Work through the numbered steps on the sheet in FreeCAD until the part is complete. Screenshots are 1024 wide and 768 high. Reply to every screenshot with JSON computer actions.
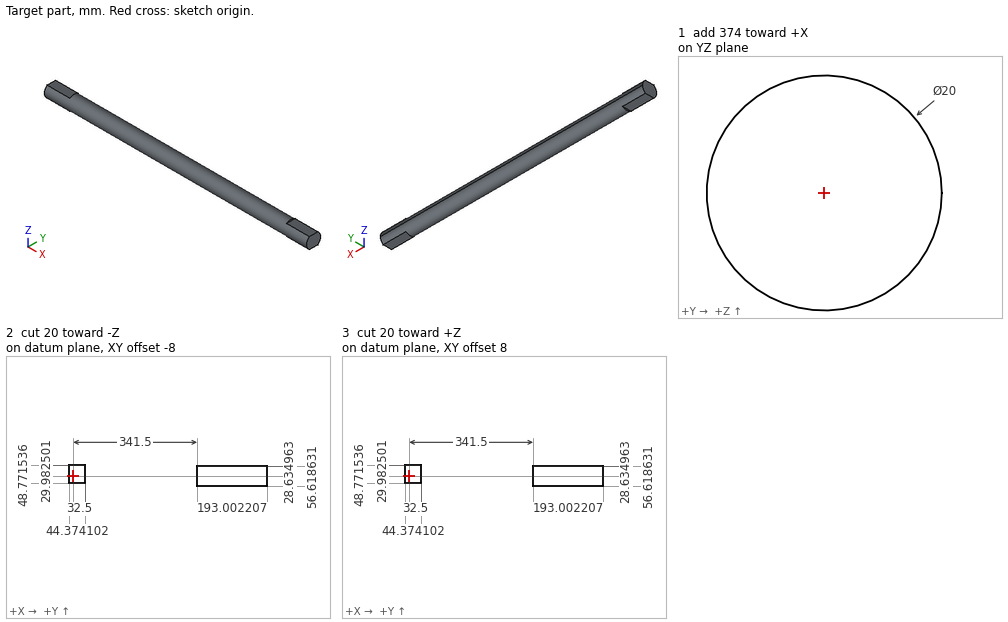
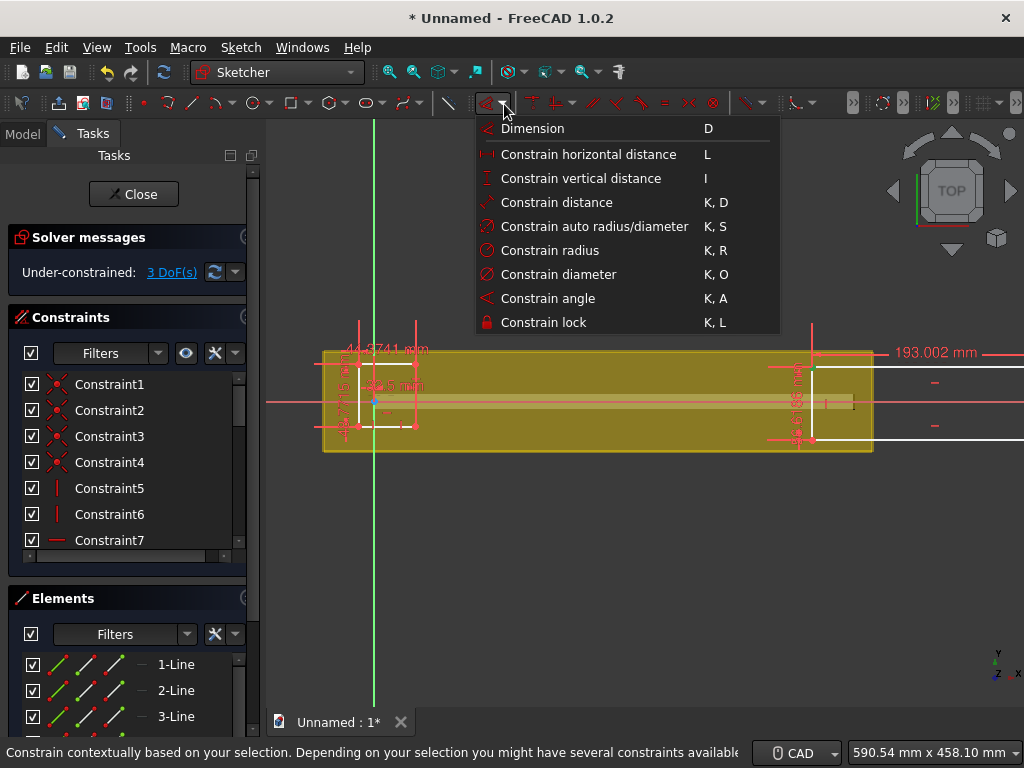
{"action": "left_click", "coordinate": [628, 154]}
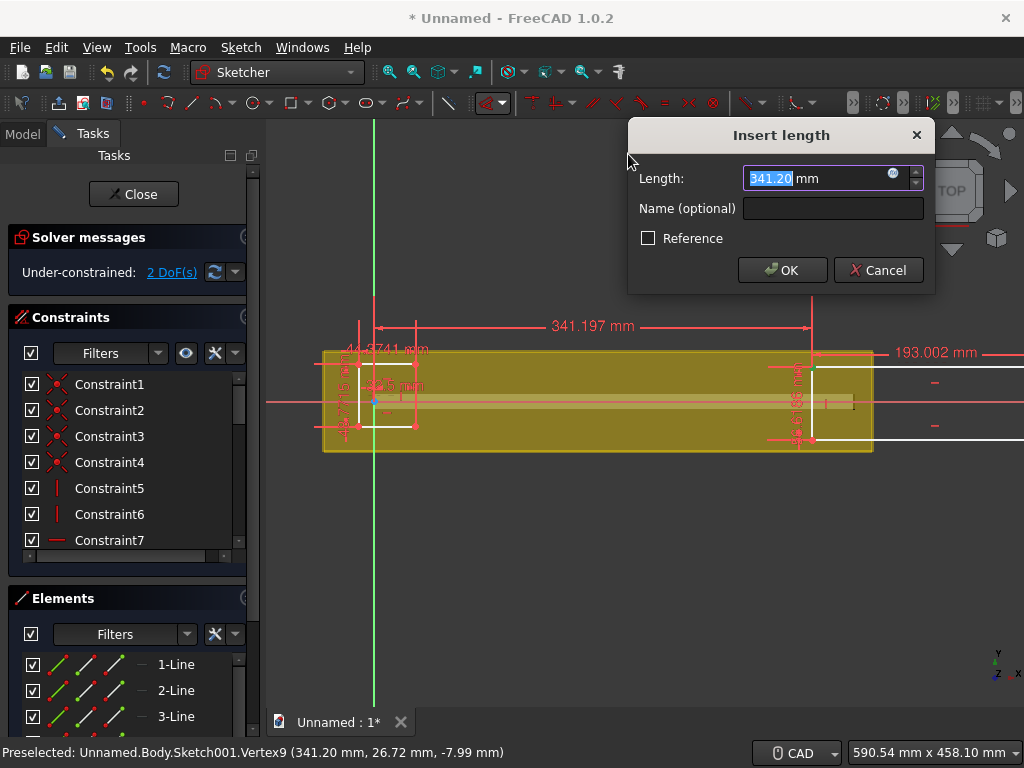
{"action": "type", "text": "341.5"}
{"action": "key", "text": "Return"}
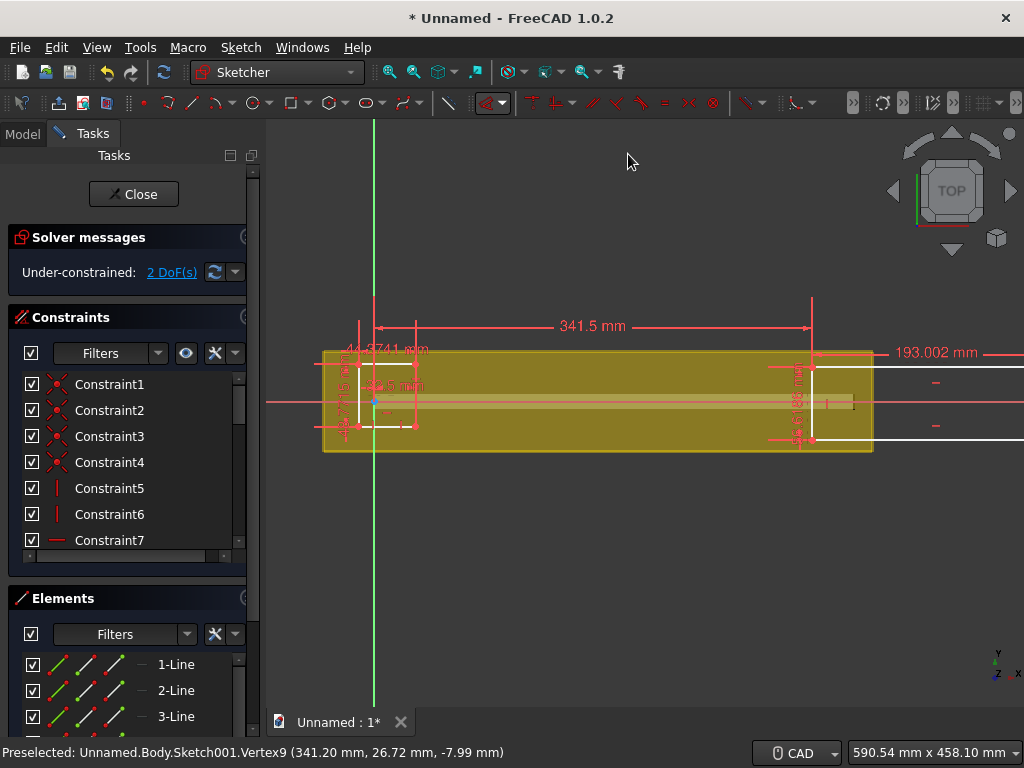
{"action": "left_click", "coordinate": [359, 364]}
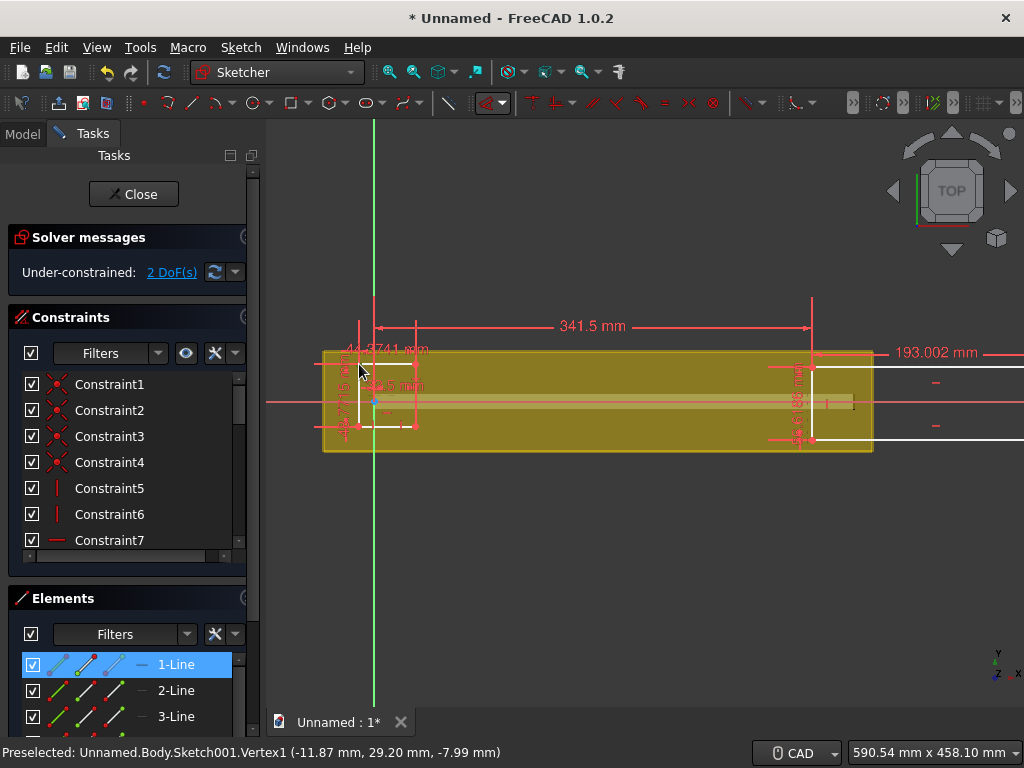
{"action": "left_click", "coordinate": [504, 104]}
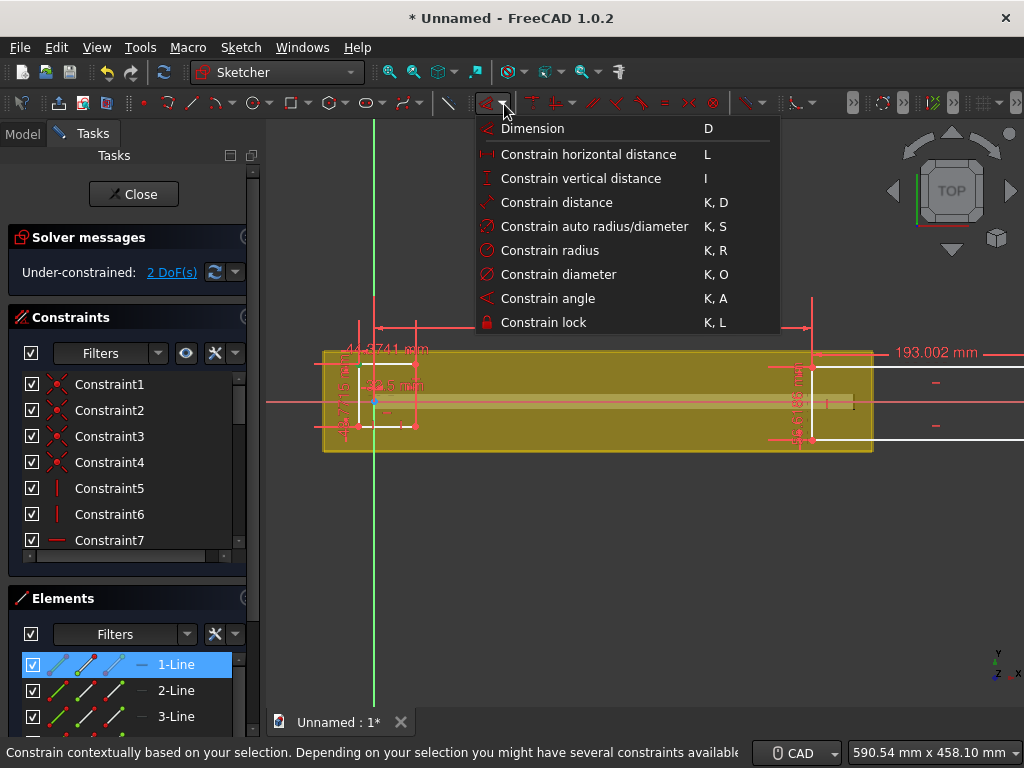
{"action": "left_click", "coordinate": [628, 178]}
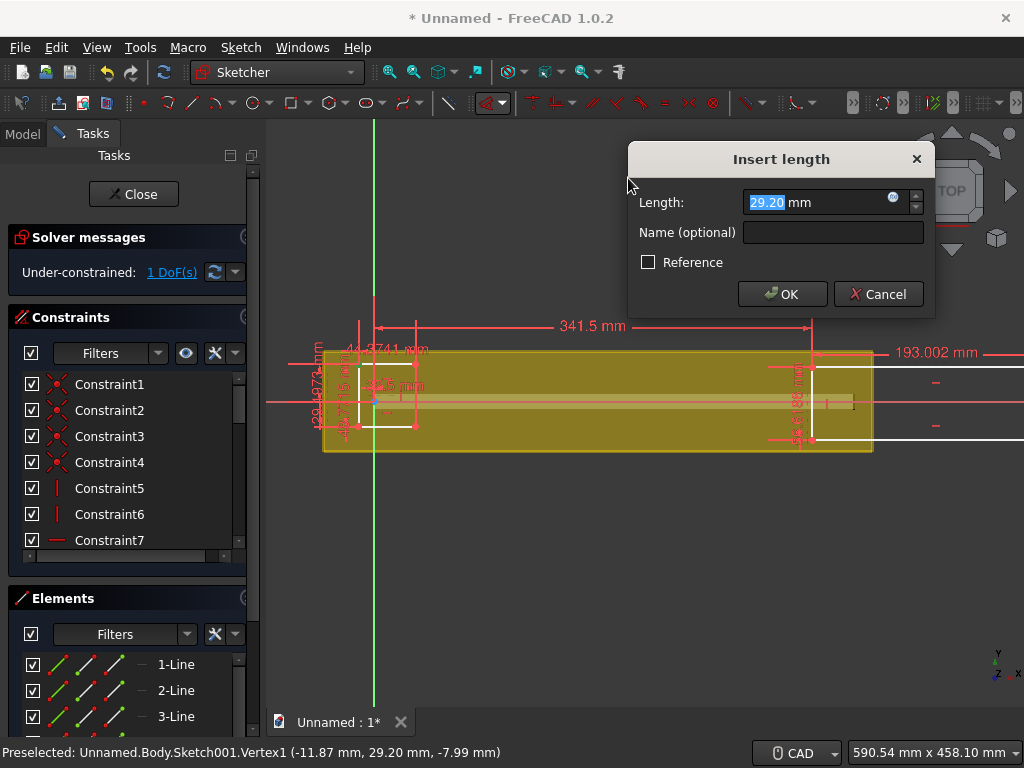
{"action": "type", "text": "29.982501"}
{"action": "key", "text": "Return"}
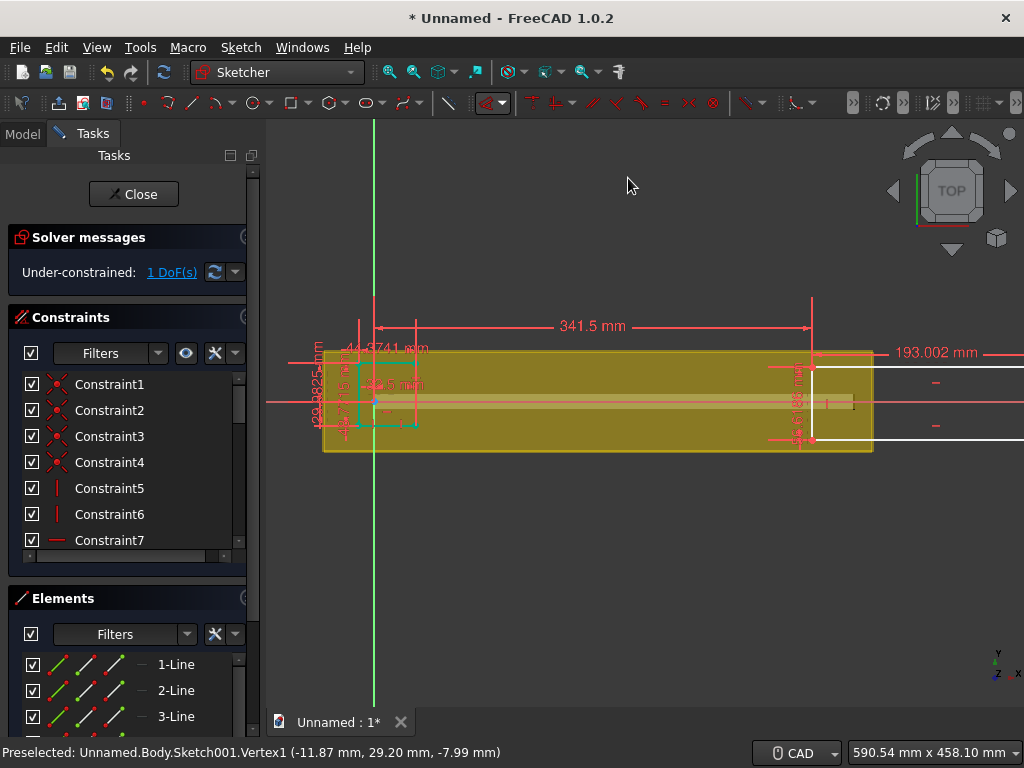
{"action": "left_click", "coordinate": [812, 367]}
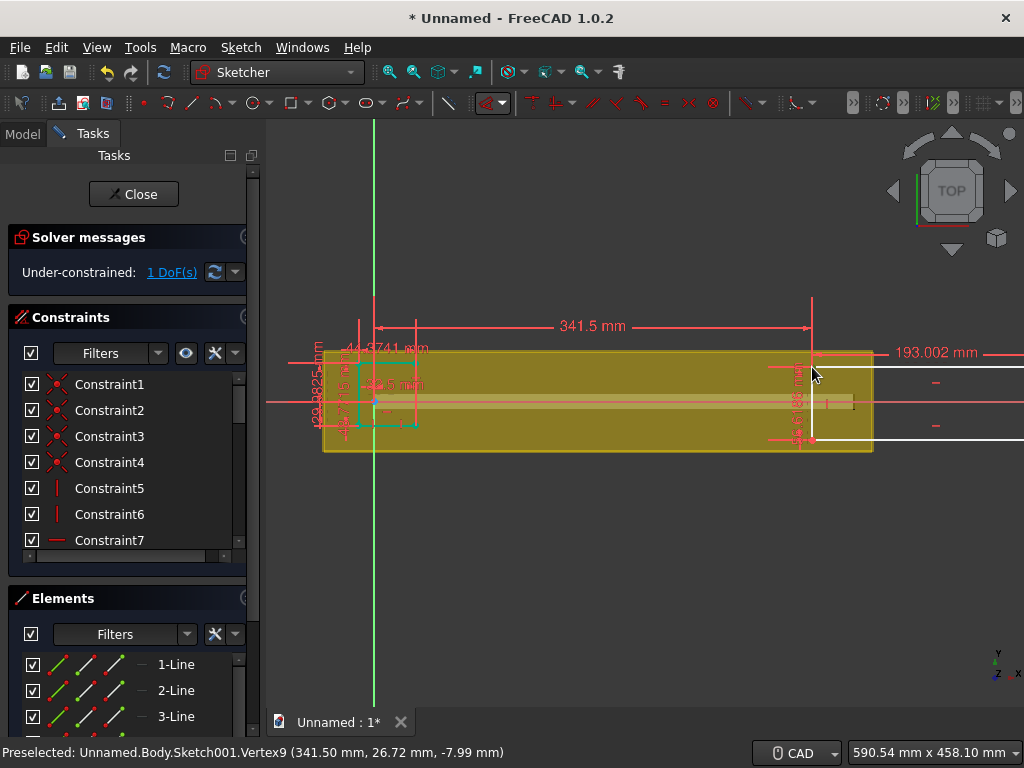
{"action": "key", "text": "i"}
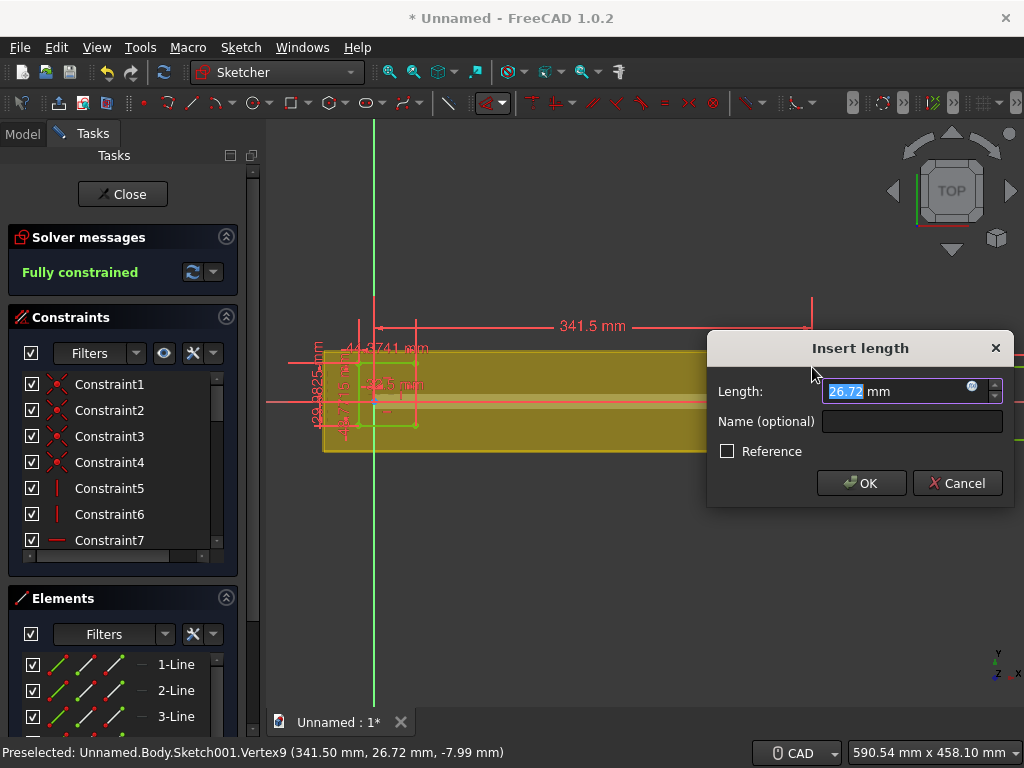
{"action": "type", "text": "28.634963"}
{"action": "key", "text": "Return"}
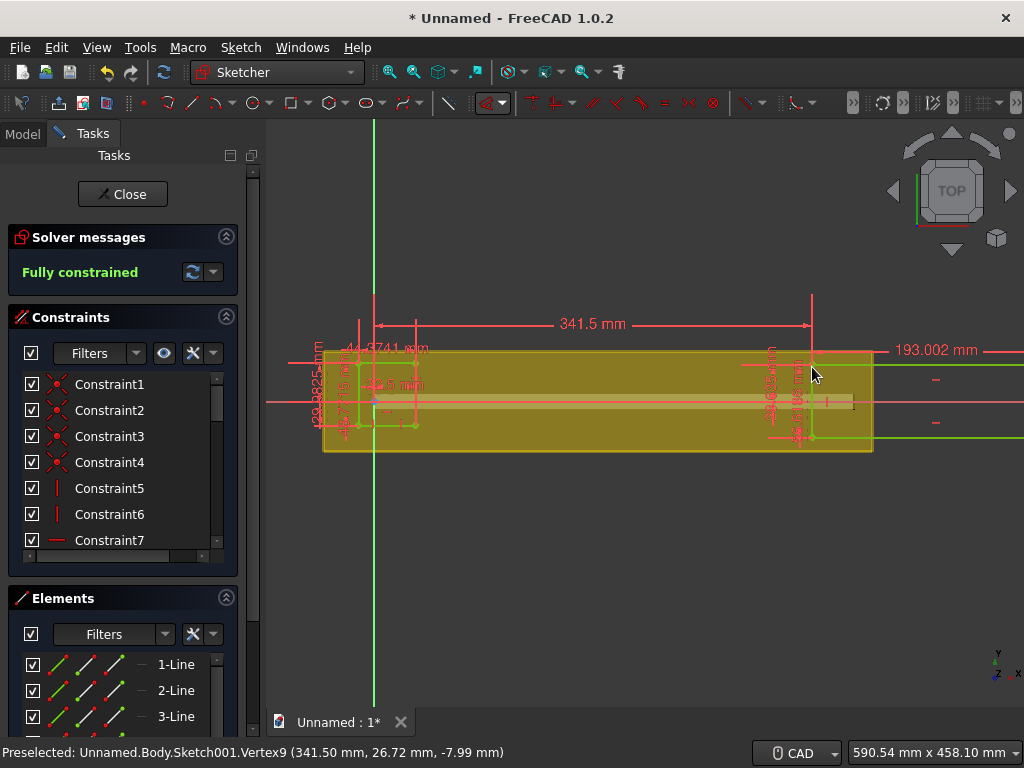
{"action": "left_click", "coordinate": [123, 194]}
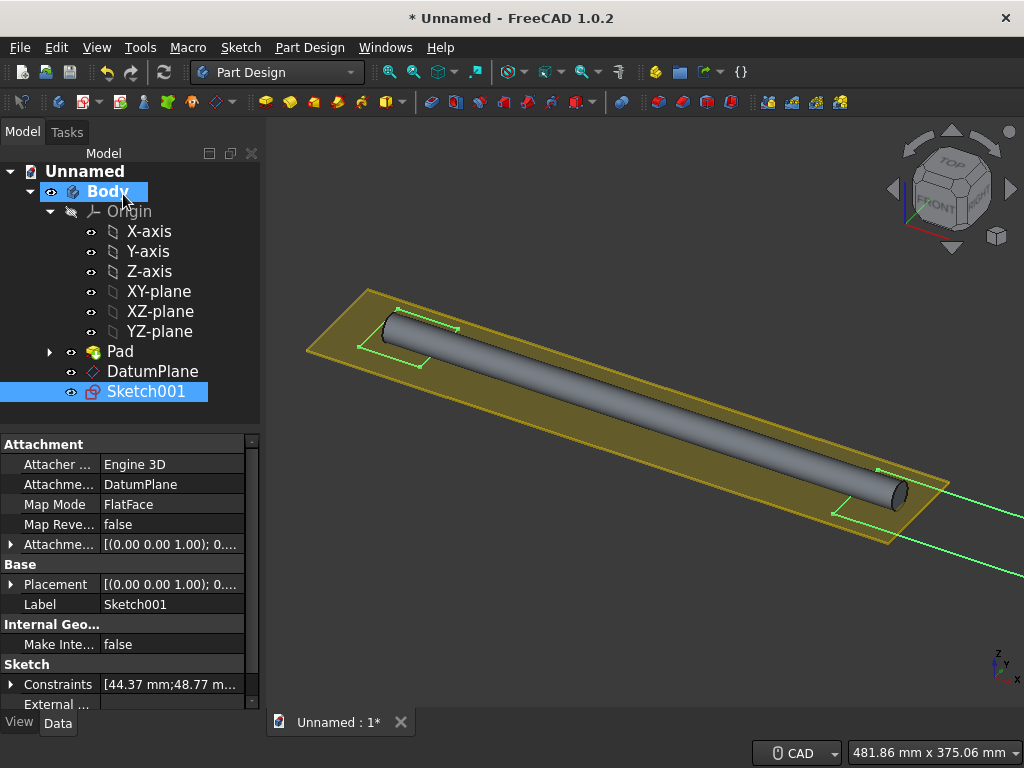
{"action": "left_click", "coordinate": [432, 102]}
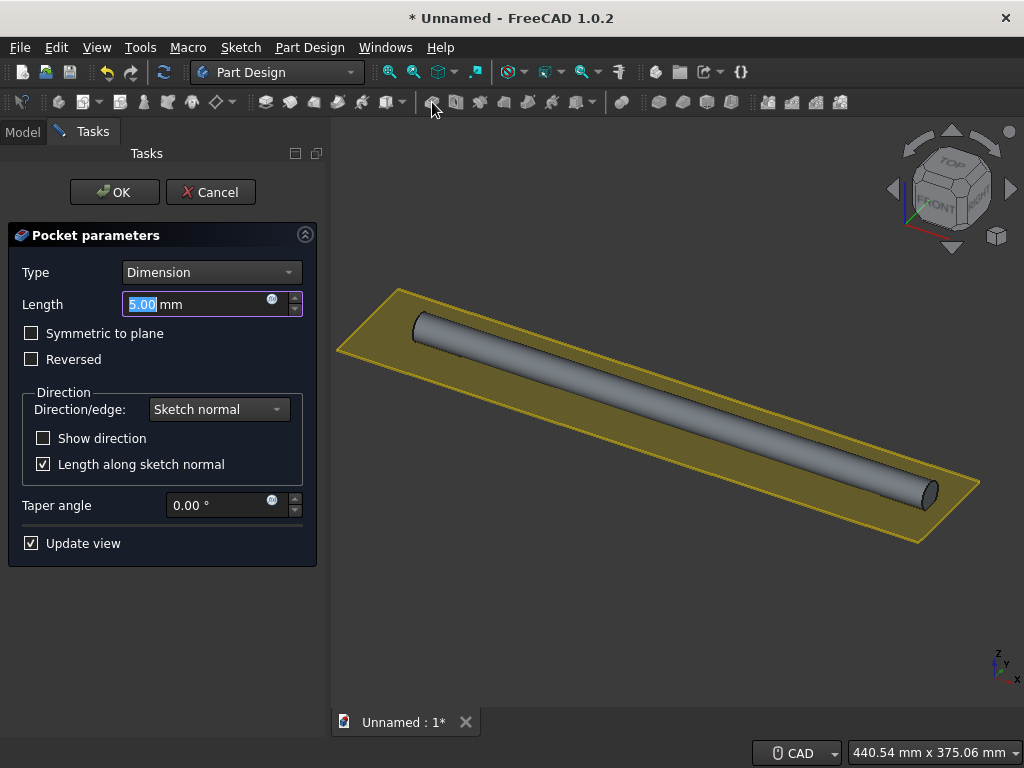
{"action": "type", "text": "20"}
{"action": "key", "text": "Tab"}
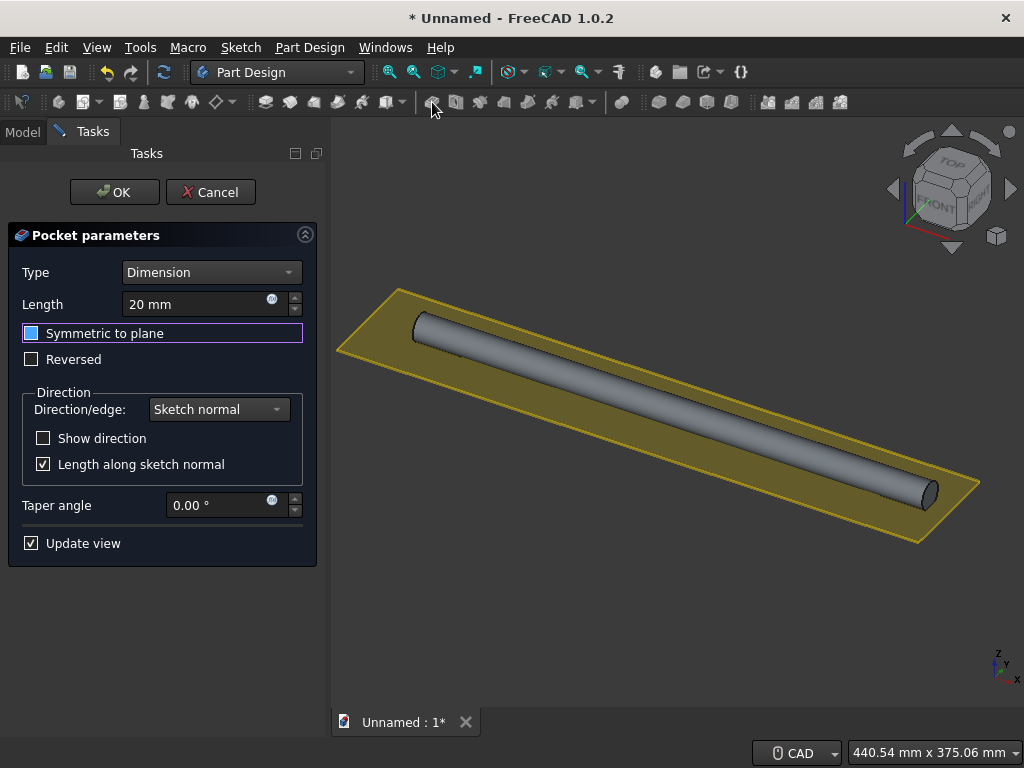
{"action": "left_click", "coordinate": [115, 192]}